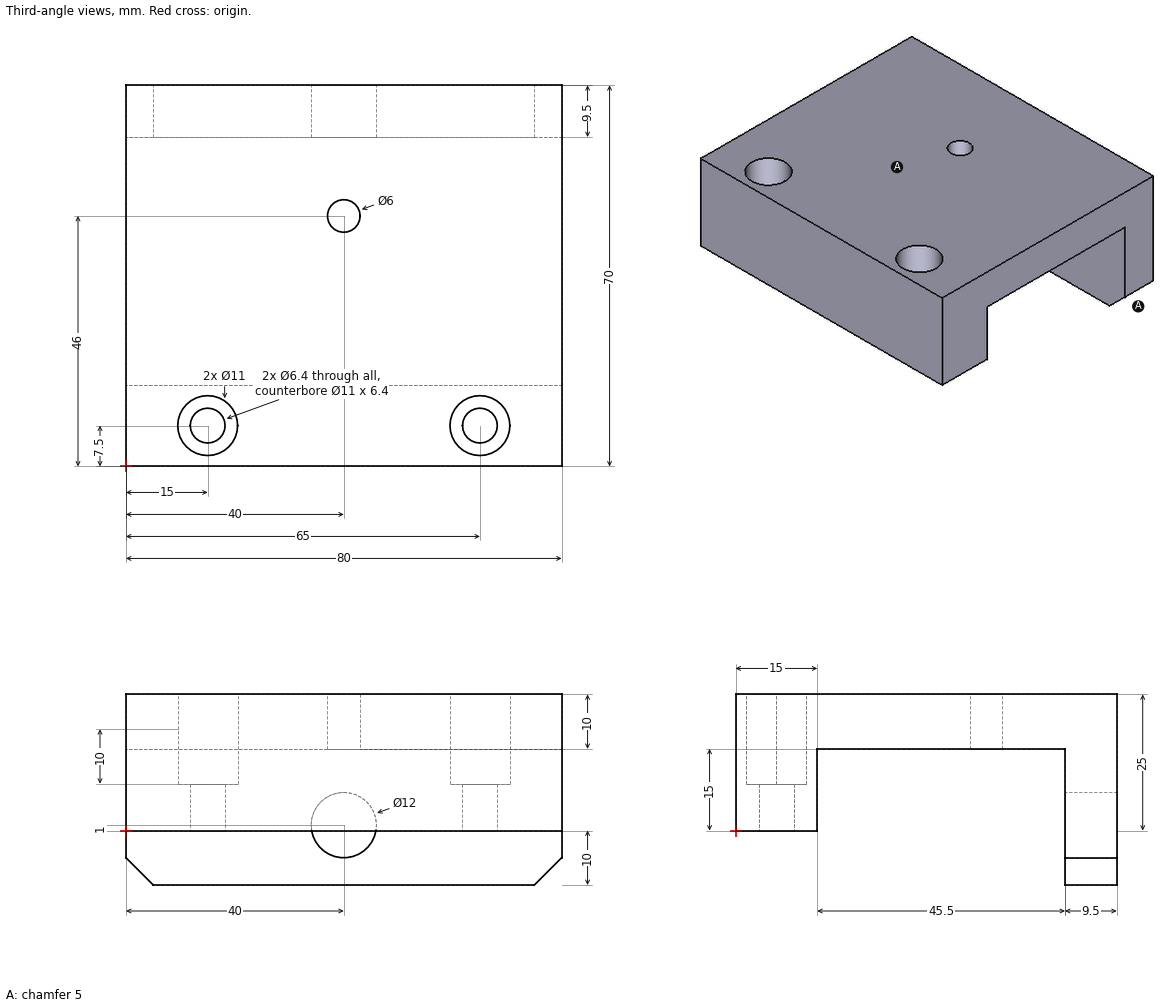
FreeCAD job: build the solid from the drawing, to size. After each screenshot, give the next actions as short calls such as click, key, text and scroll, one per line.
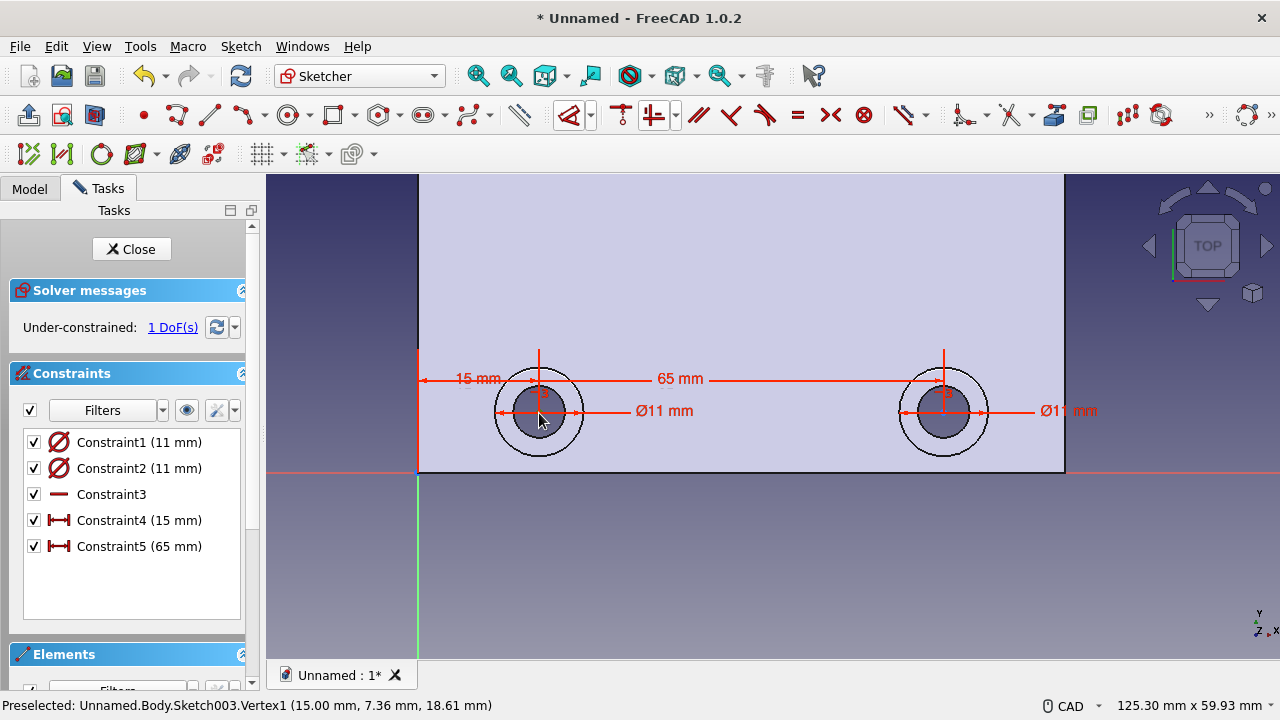
key(i)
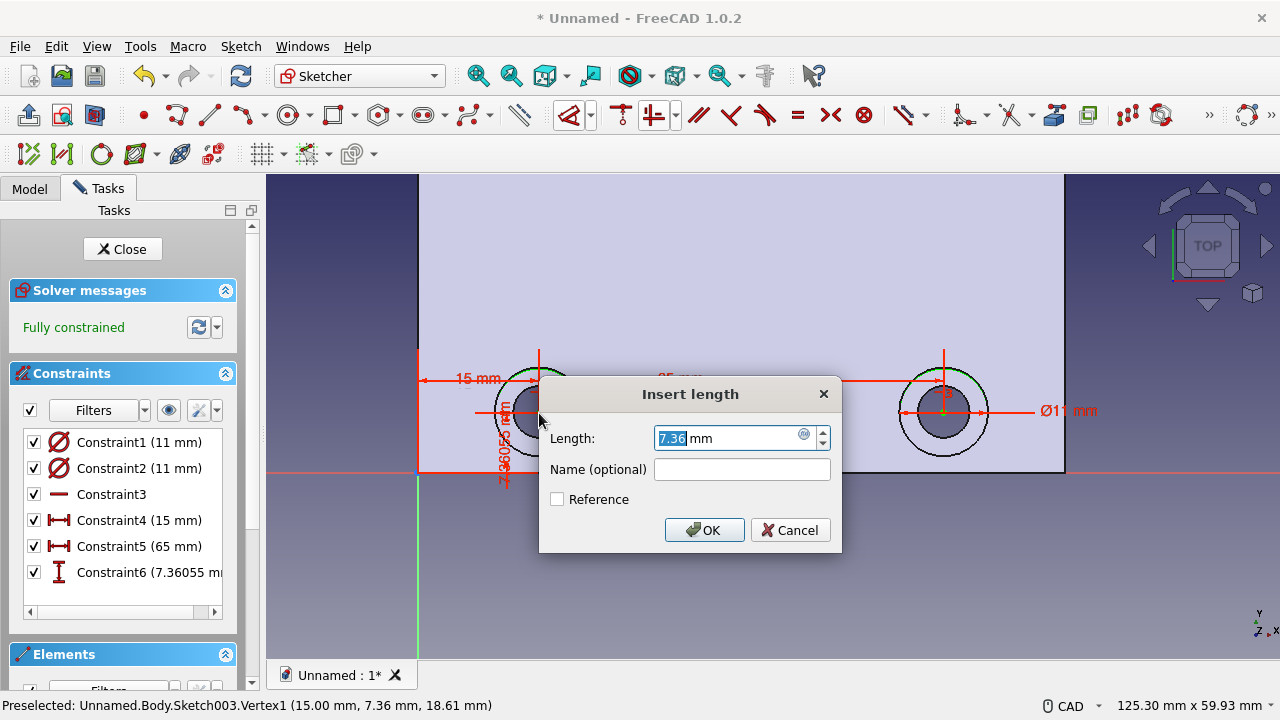
text(7.5)
key(Return)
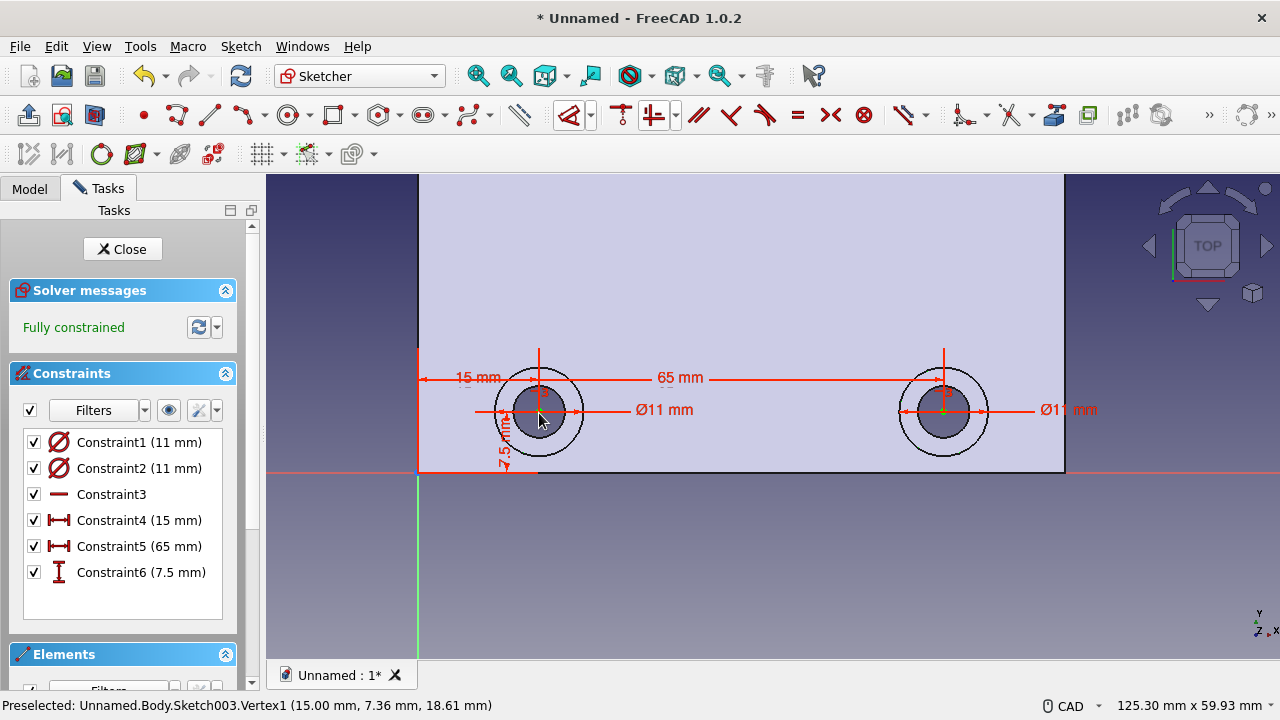
click(123, 249)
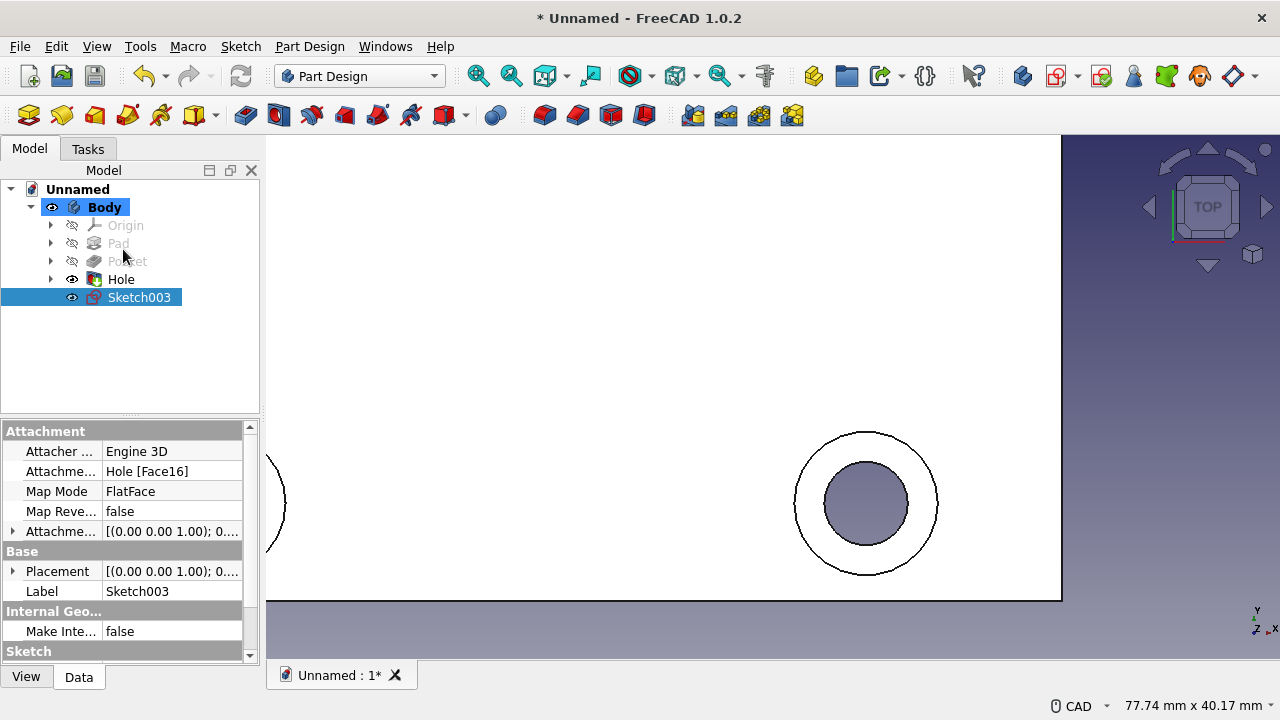
click(246, 116)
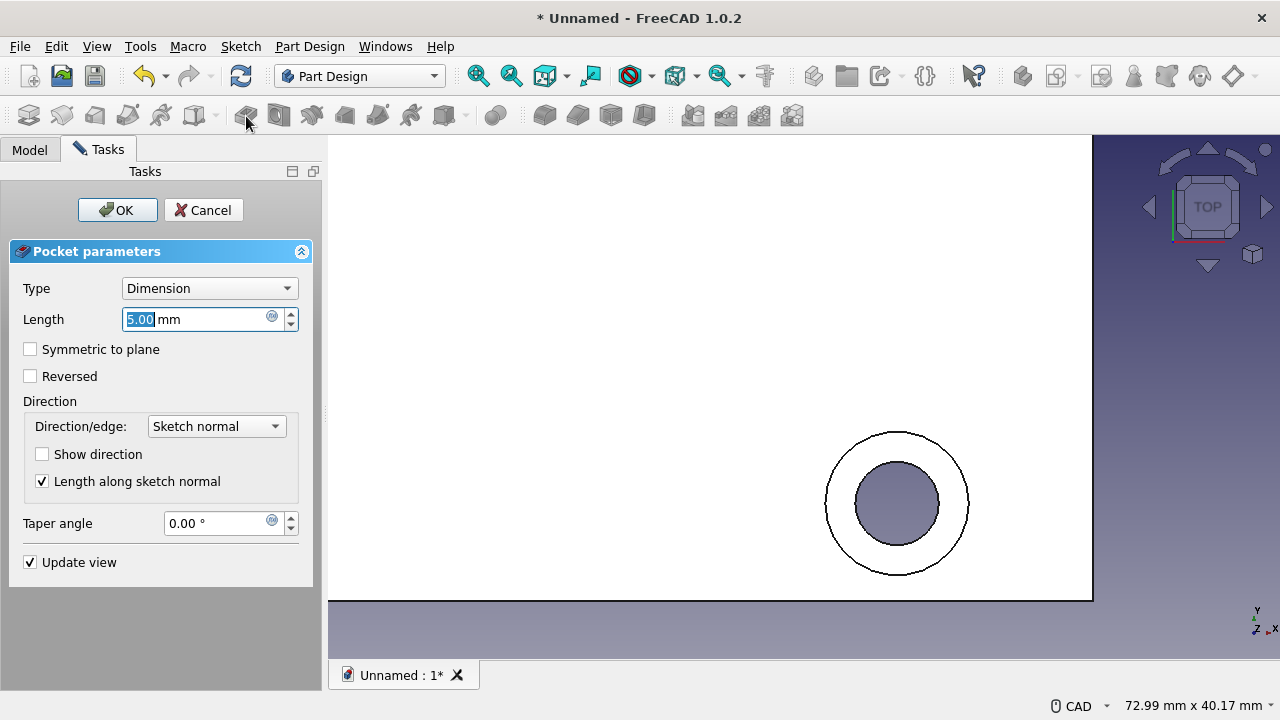
text(10)
key(Tab)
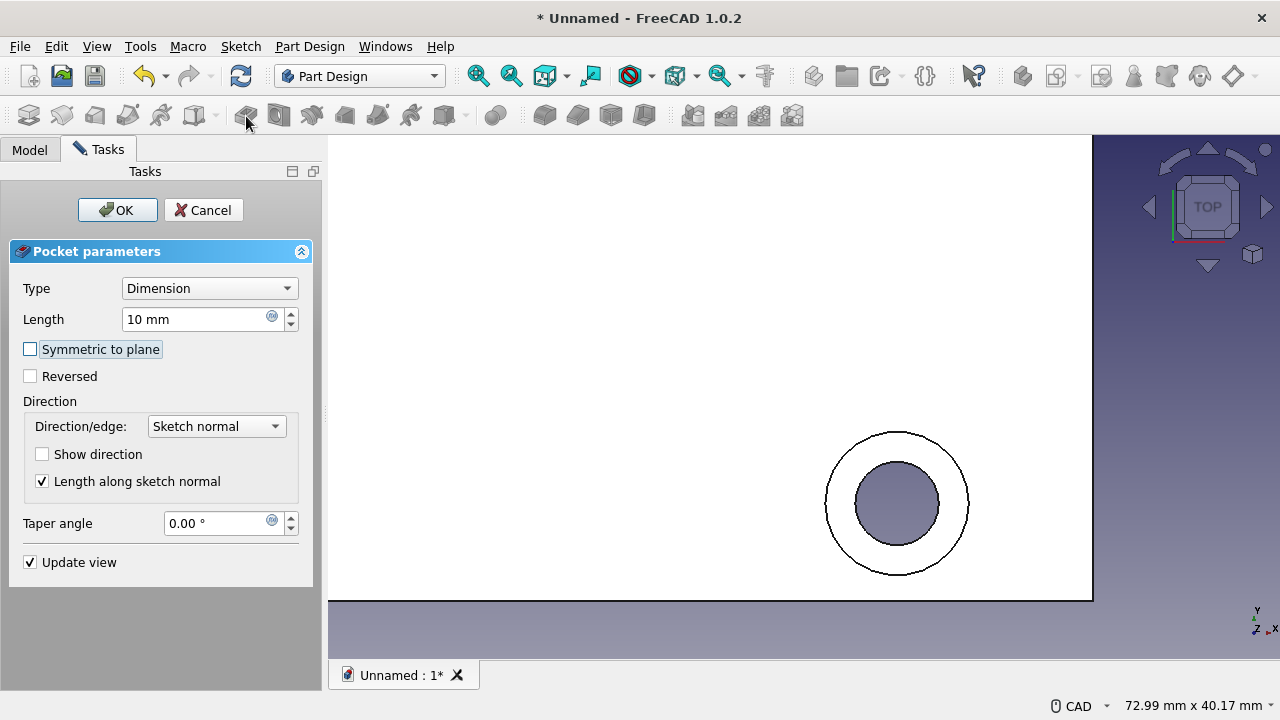
click(118, 210)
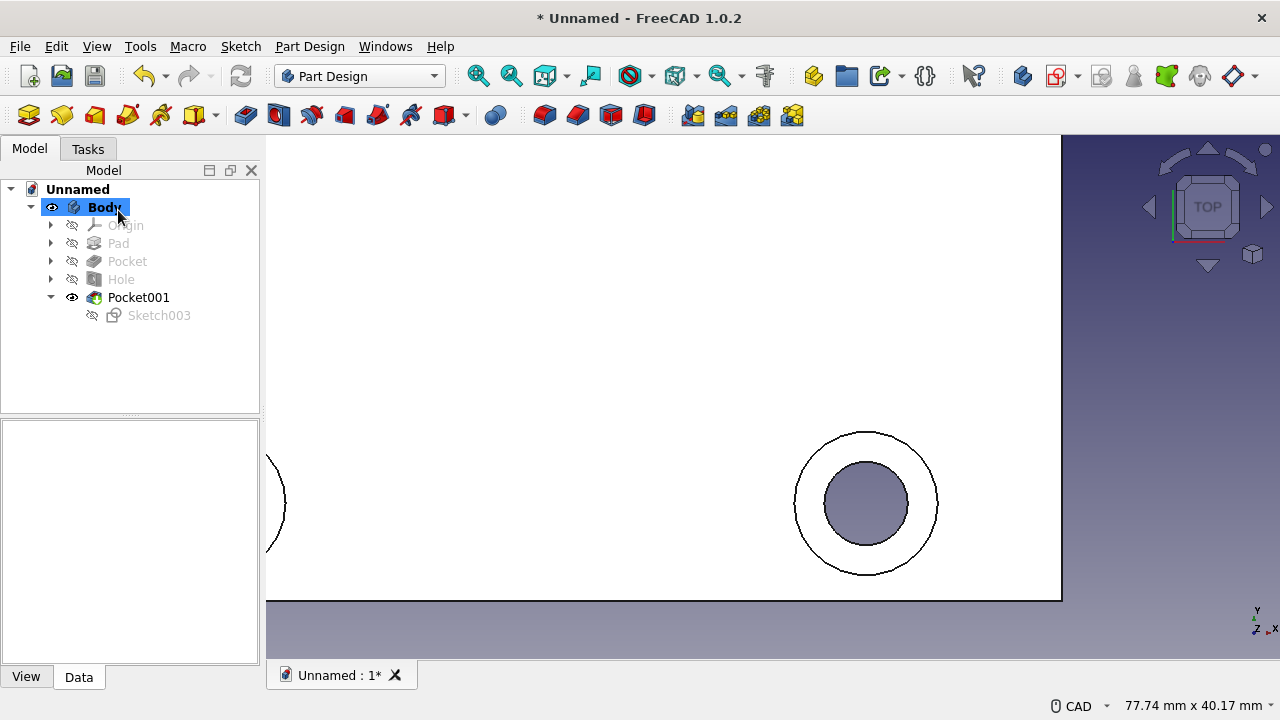
click(479, 76)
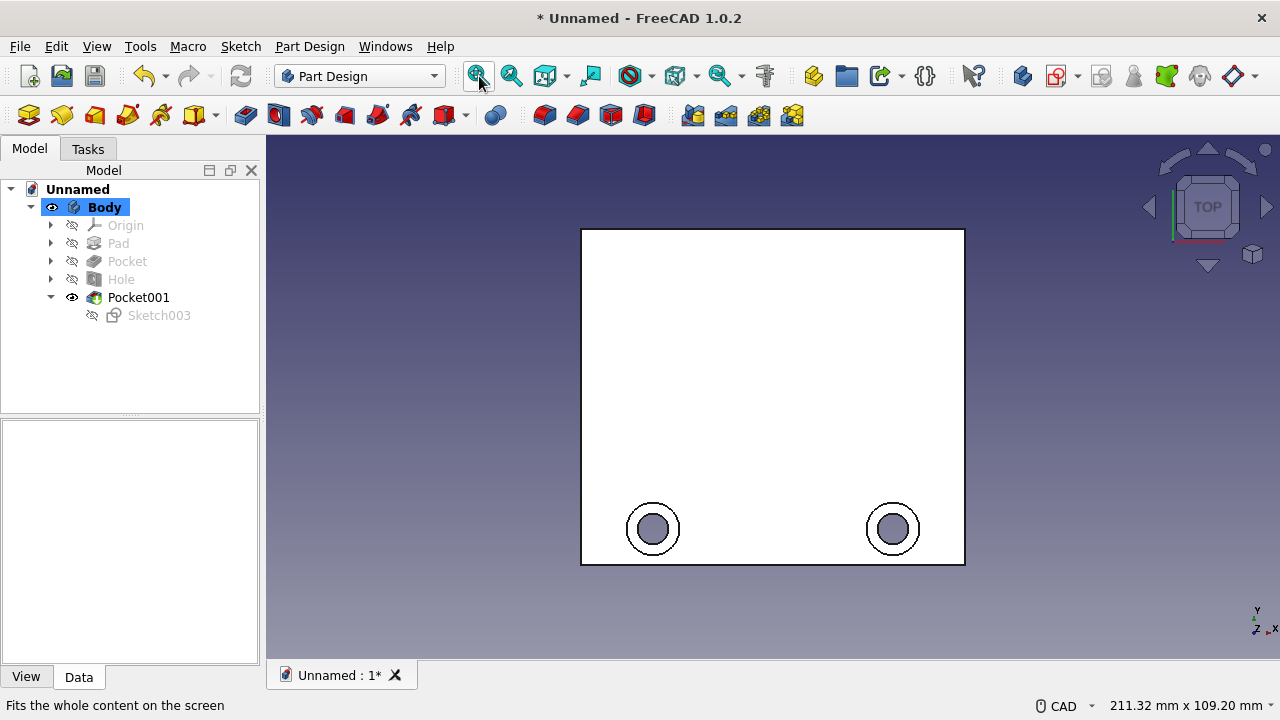
click(773, 396)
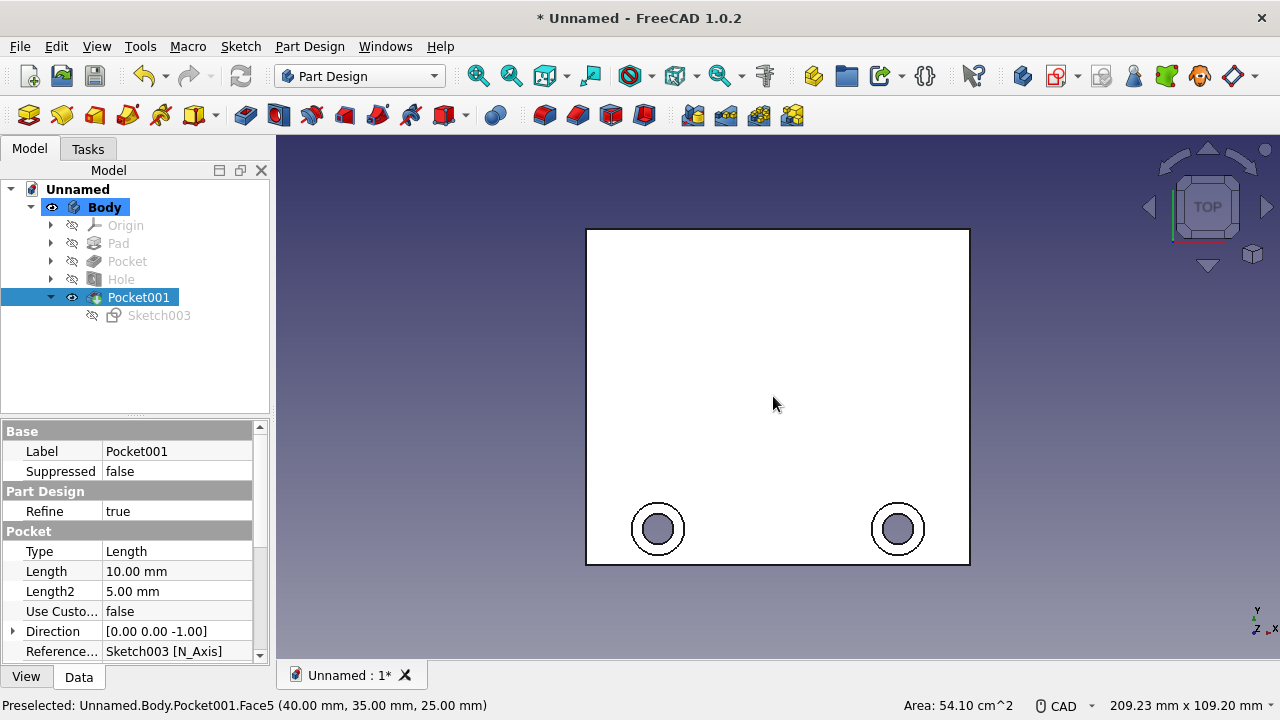
click(1056, 76)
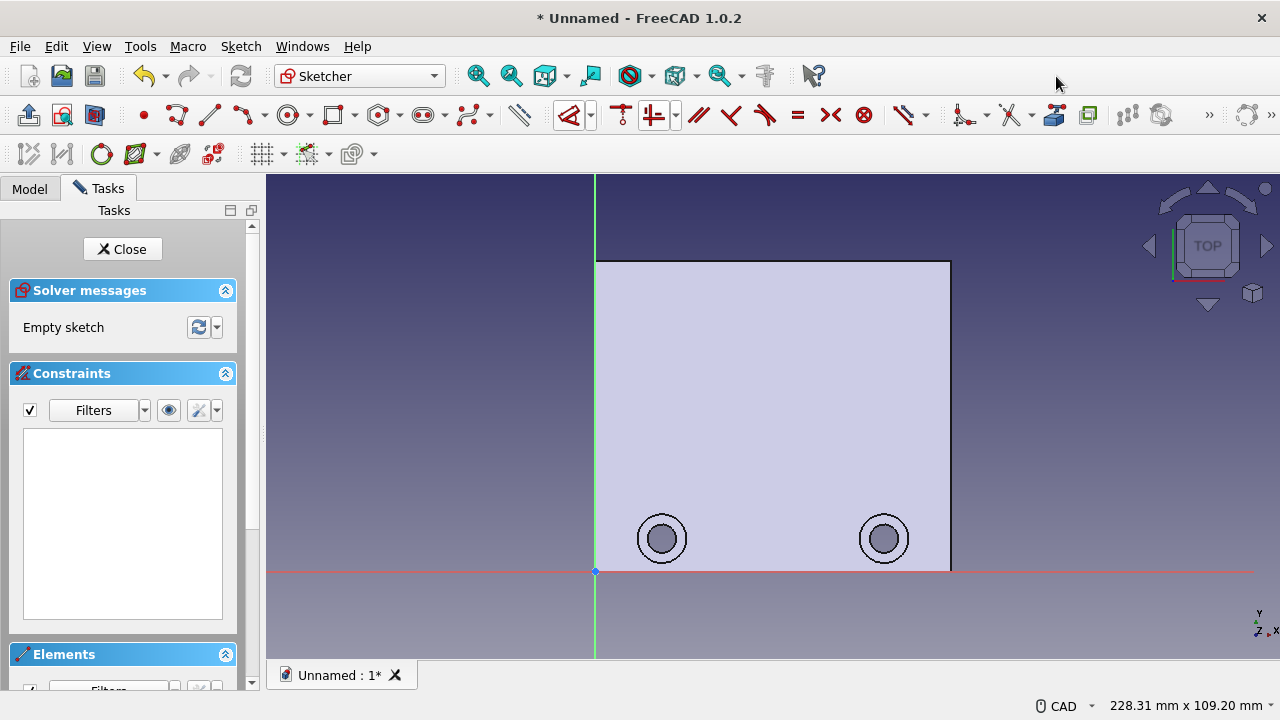
scroll(780, 363, up, 12)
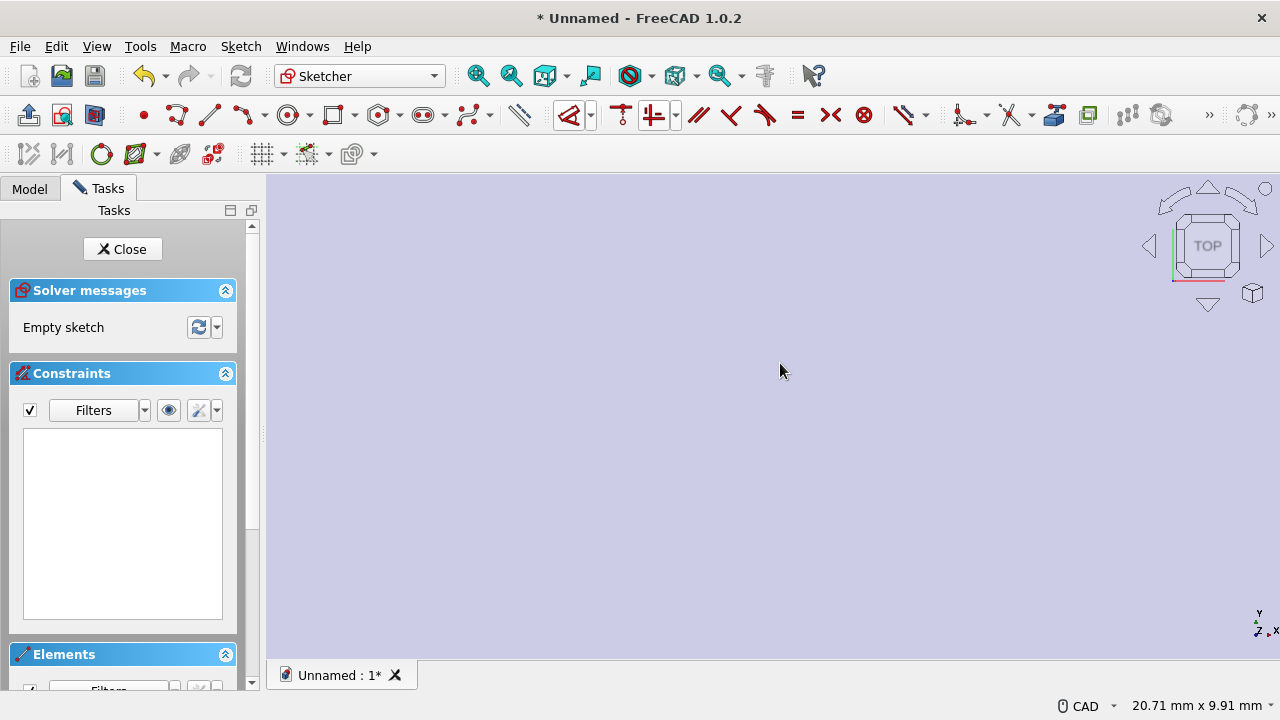
click(288, 116)